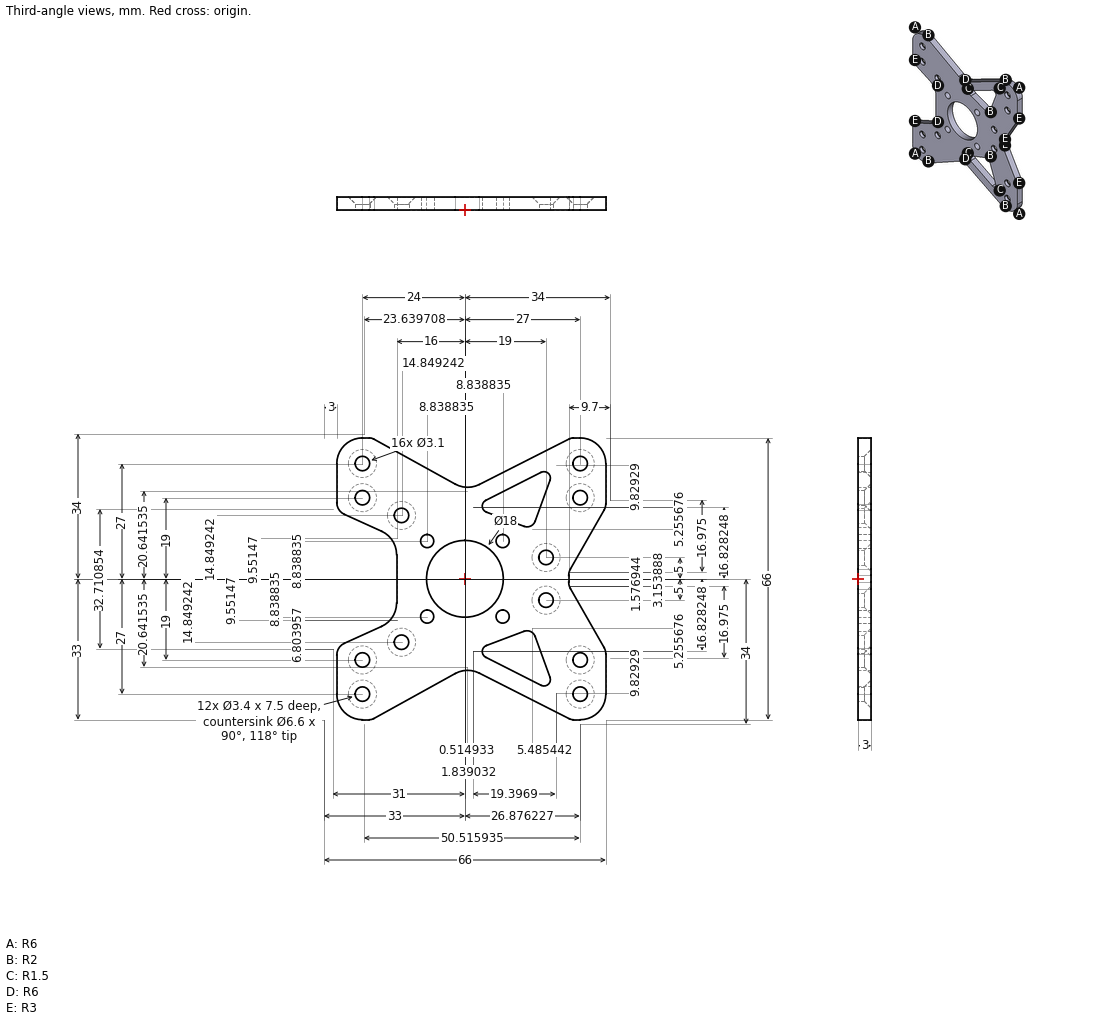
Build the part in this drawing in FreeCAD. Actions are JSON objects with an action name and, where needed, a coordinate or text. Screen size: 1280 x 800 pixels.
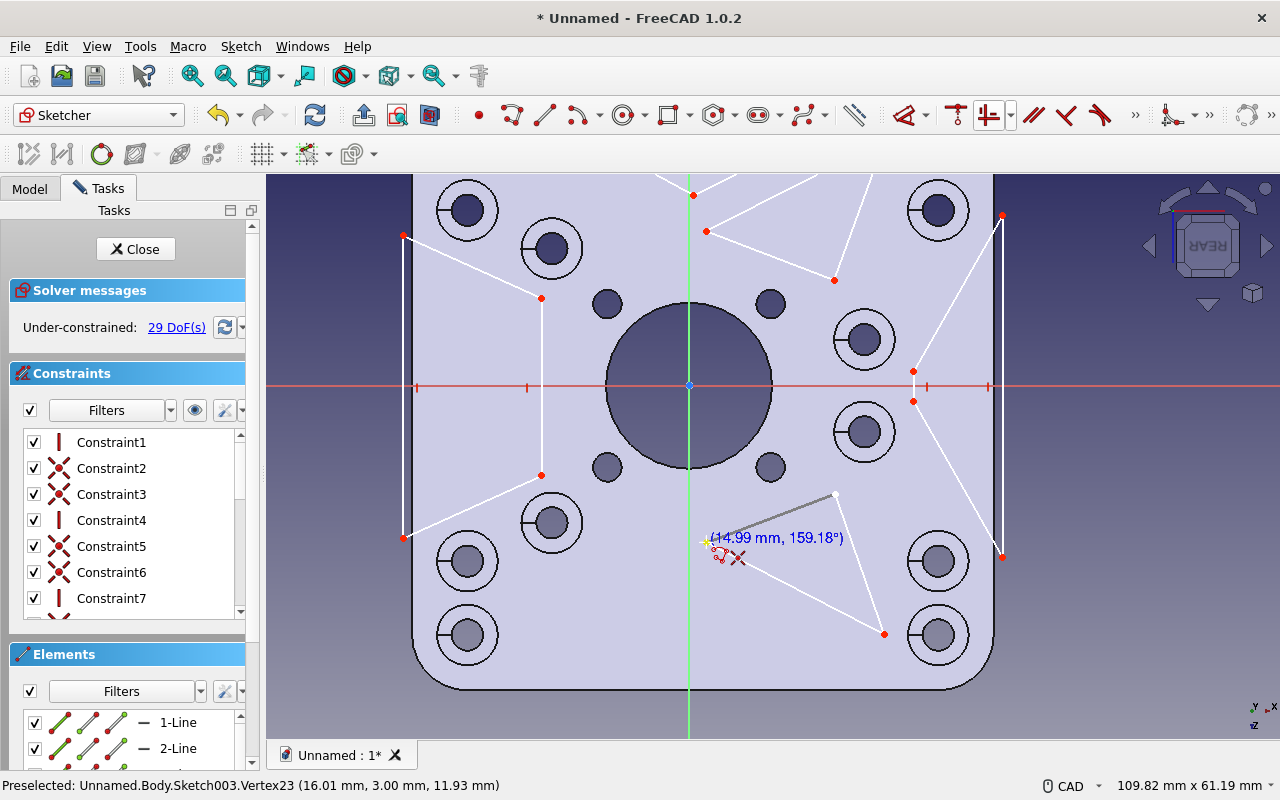
{"action": "left_click", "coordinate": [706, 542]}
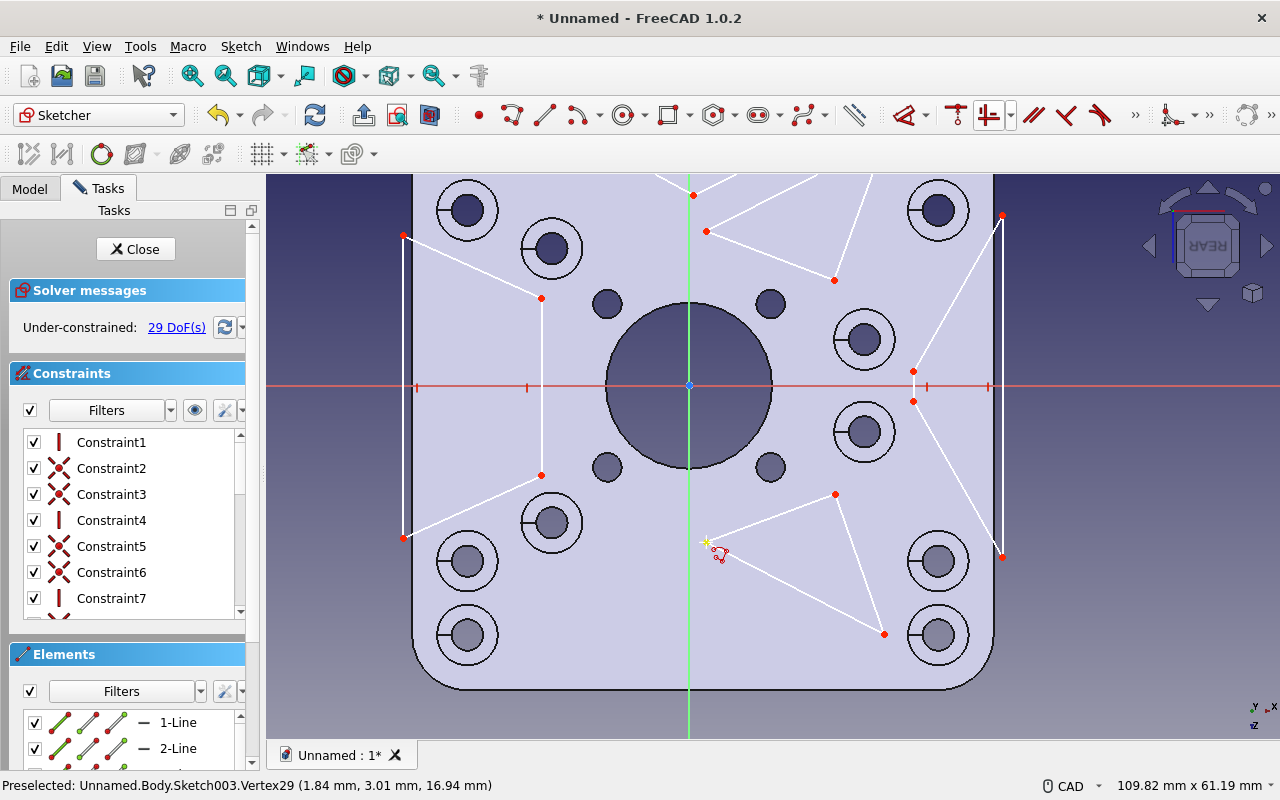
{"action": "scroll", "coordinate": [694, 576], "scroll_direction": "up", "scroll_amount": 7}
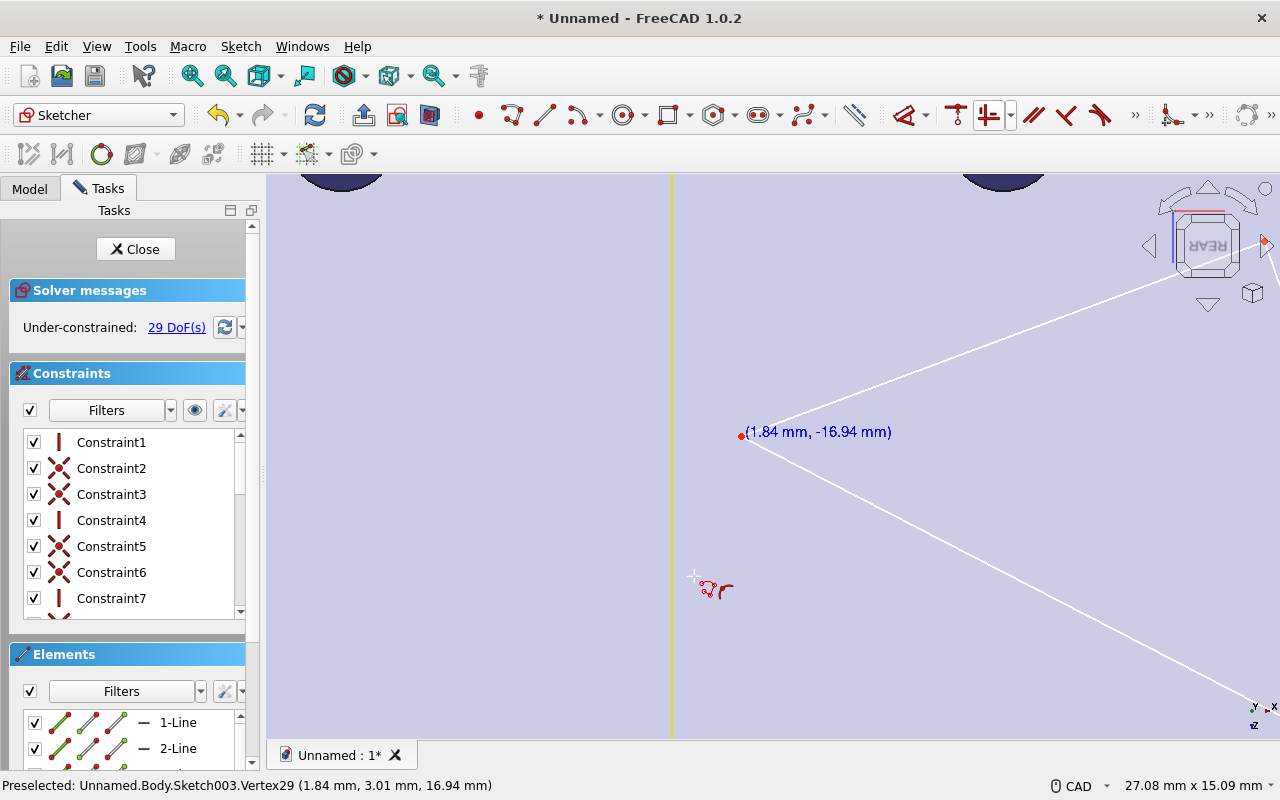
{"action": "left_click", "coordinate": [692, 575]}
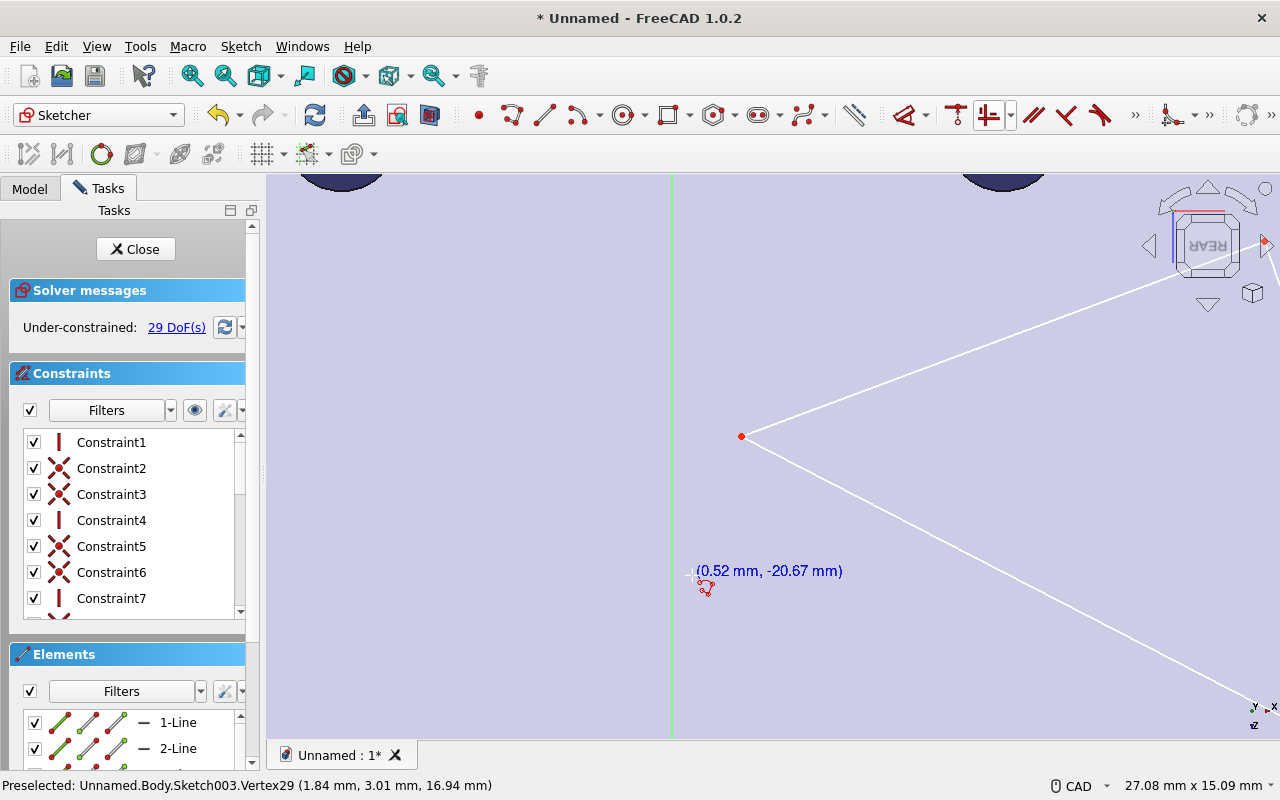
{"action": "scroll", "coordinate": [701, 559], "scroll_direction": "down", "scroll_amount": 10}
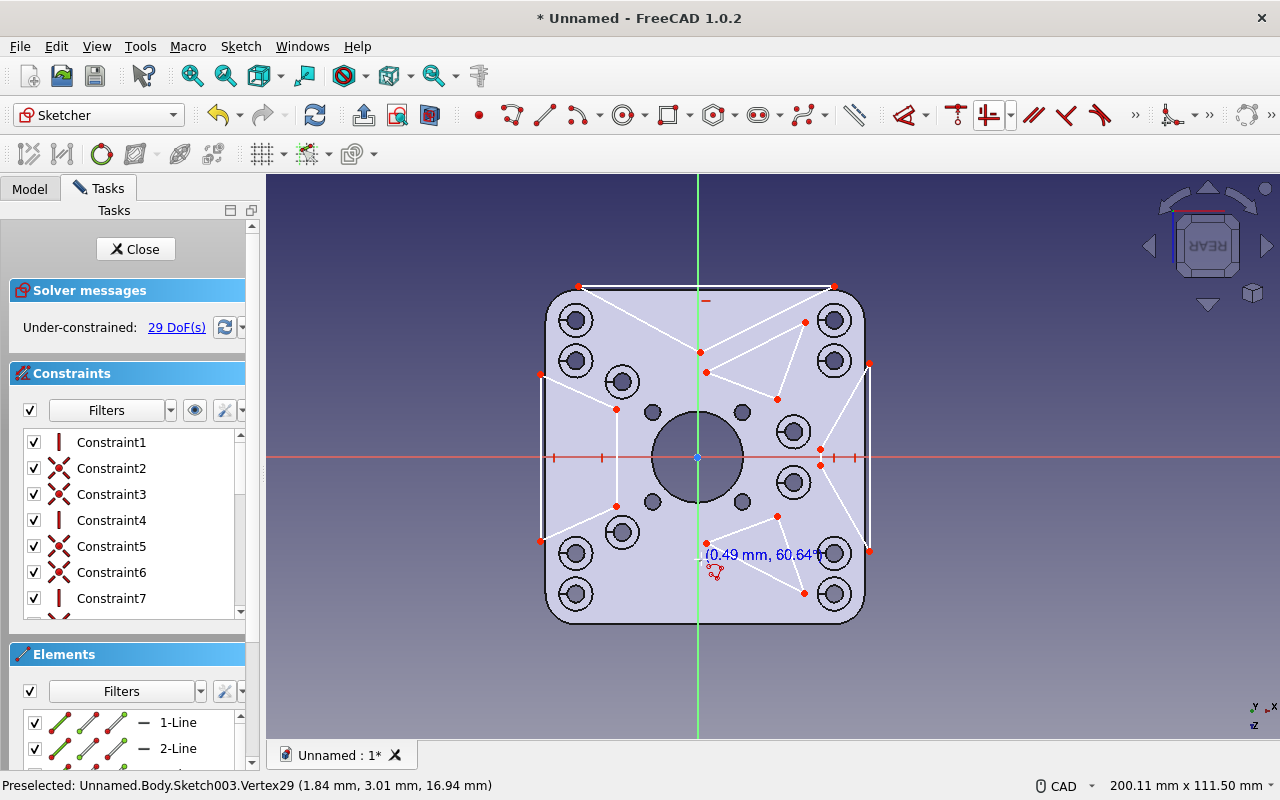
{"action": "left_click", "coordinate": [578, 629]}
{"action": "left_click", "coordinate": [834, 629]}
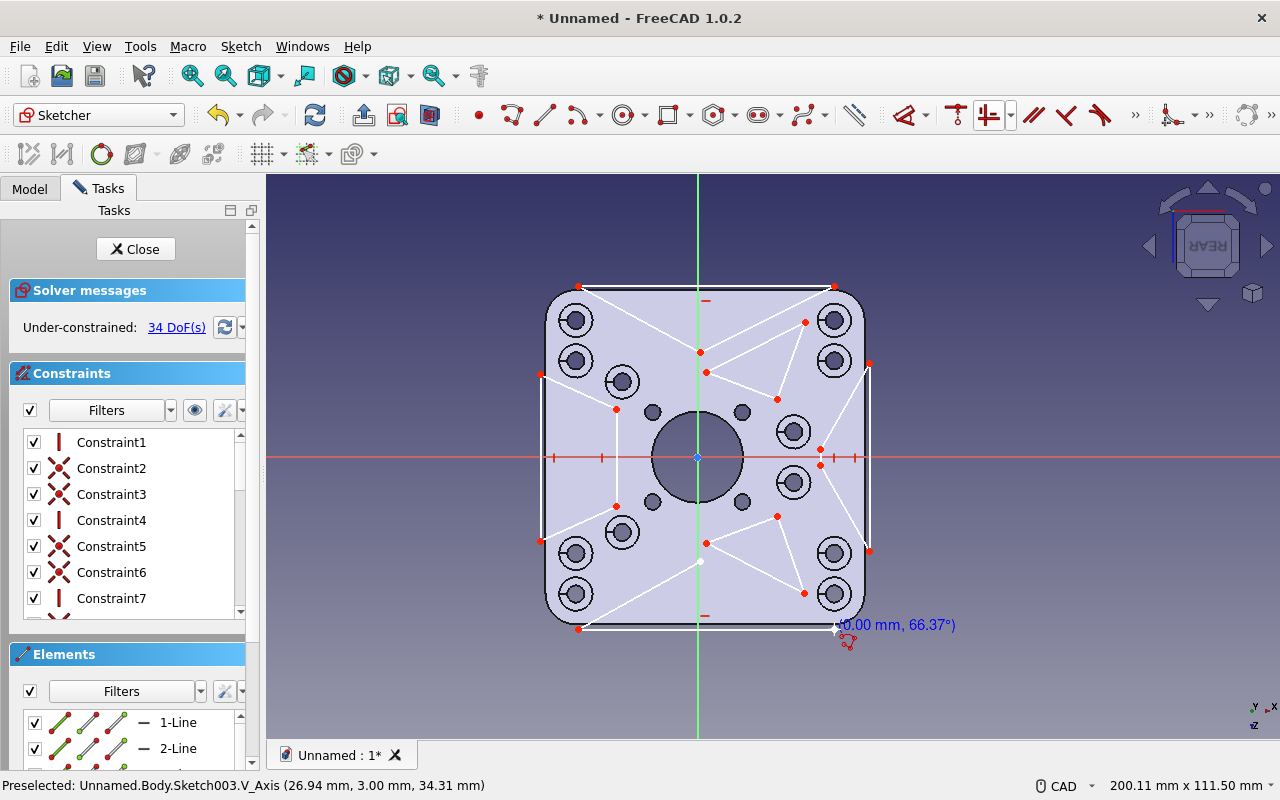
{"action": "scroll", "coordinate": [700, 562], "scroll_direction": "up", "scroll_amount": 10}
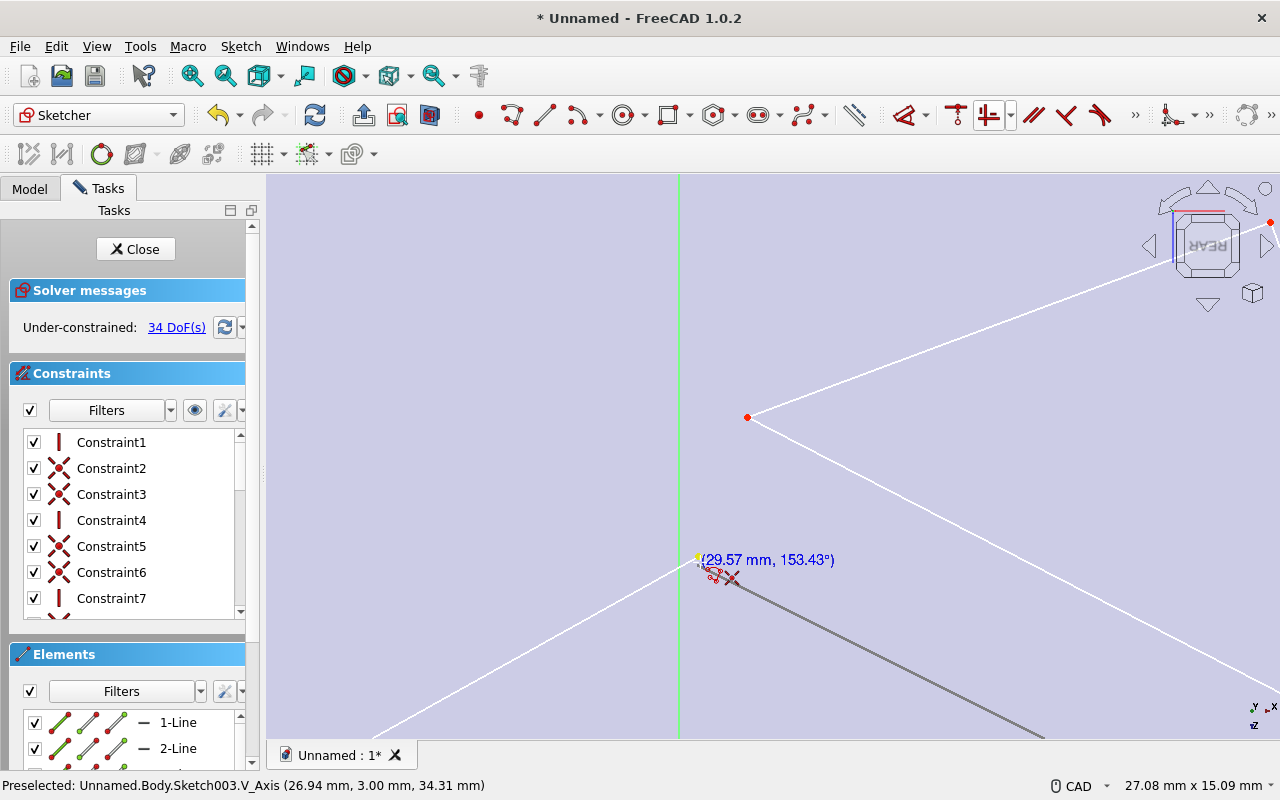
{"action": "left_click", "coordinate": [698, 557]}
{"action": "key", "text": "Escape"}
{"action": "key", "text": "Escape"}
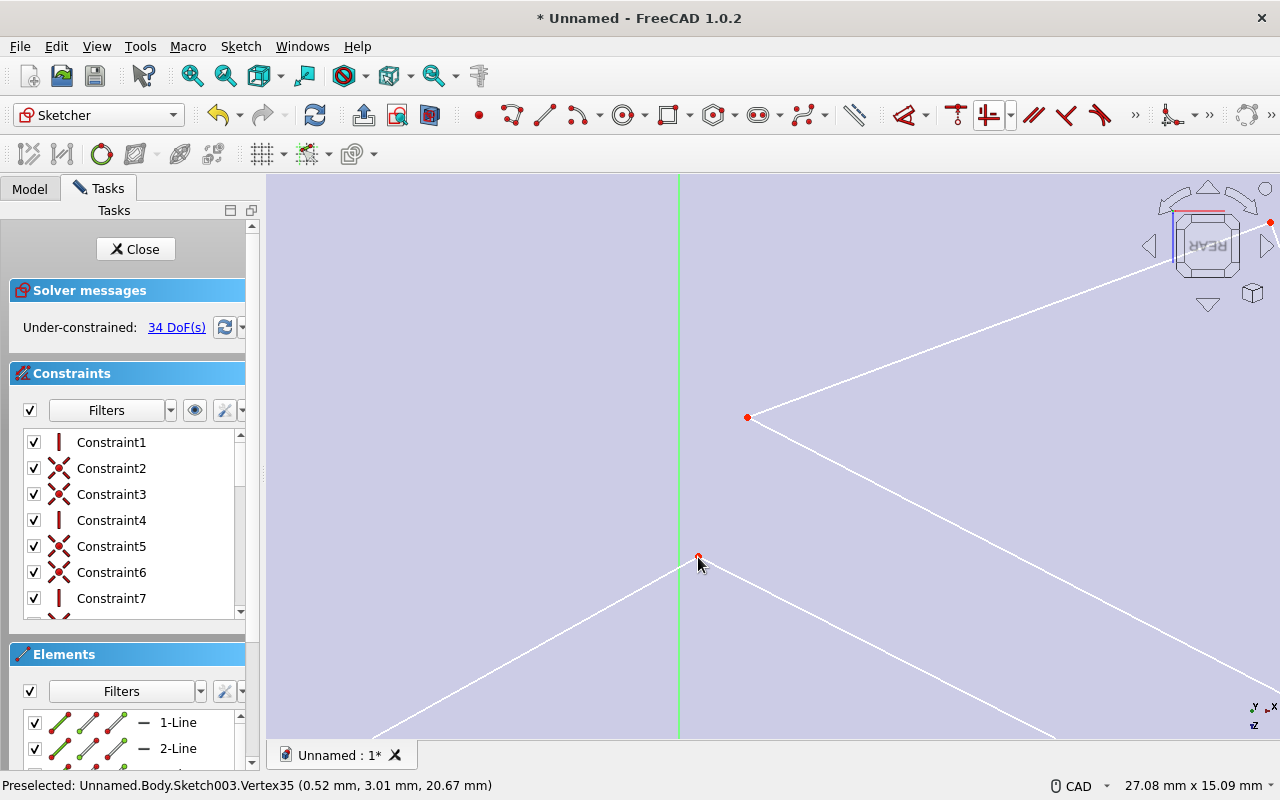
{"action": "left_click", "coordinate": [904, 116]}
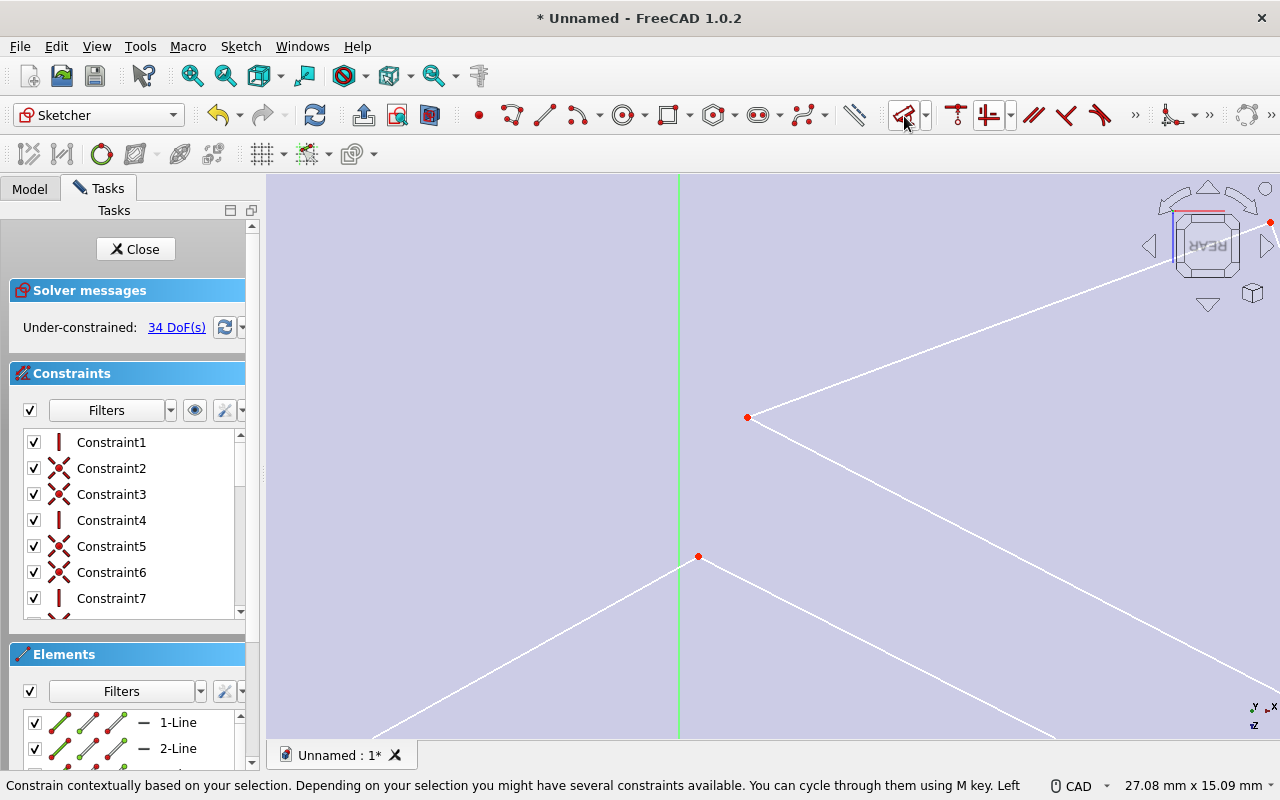
{"action": "scroll", "coordinate": [700, 562], "scroll_direction": "down", "scroll_amount": 10}